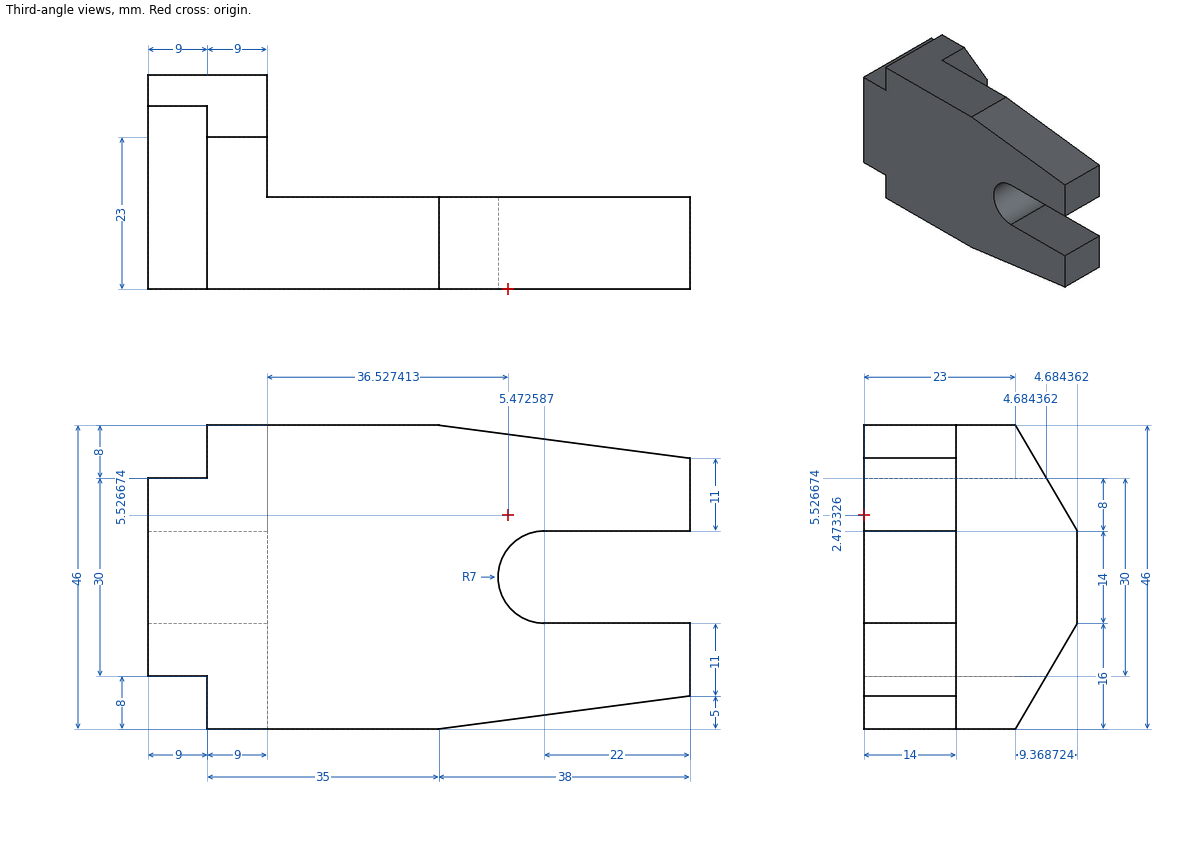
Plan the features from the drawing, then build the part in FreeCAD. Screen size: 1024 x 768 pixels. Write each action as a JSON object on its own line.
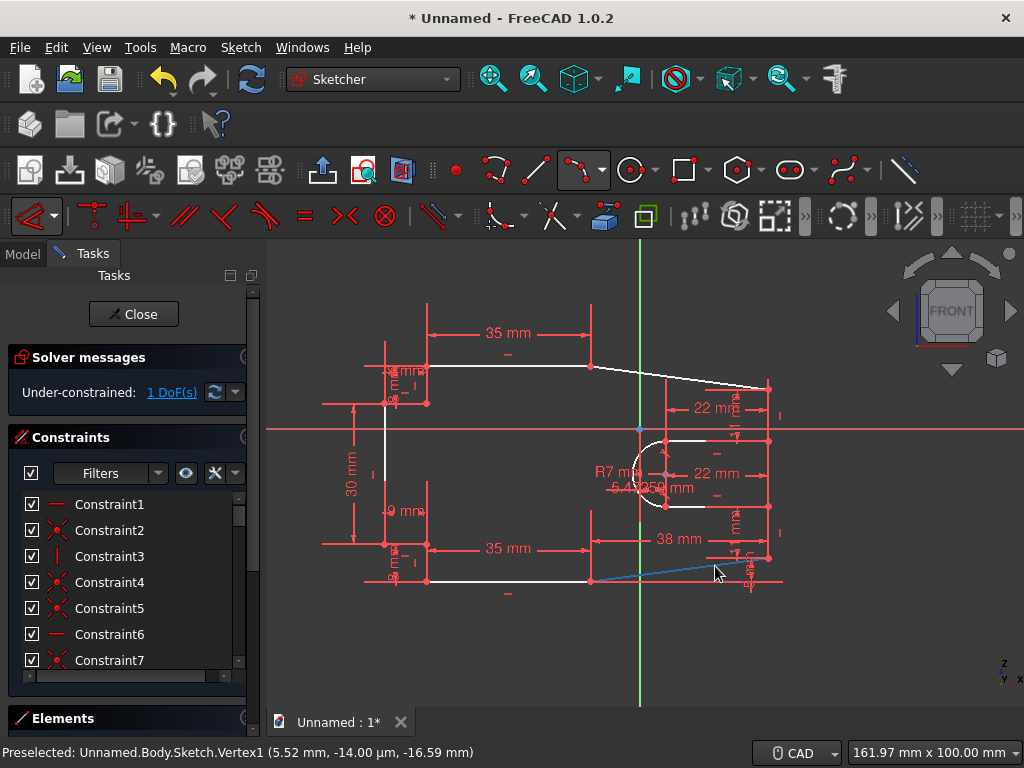
{"action": "scroll", "coordinate": [385, 404], "scroll_direction": "up", "scroll_amount": 3}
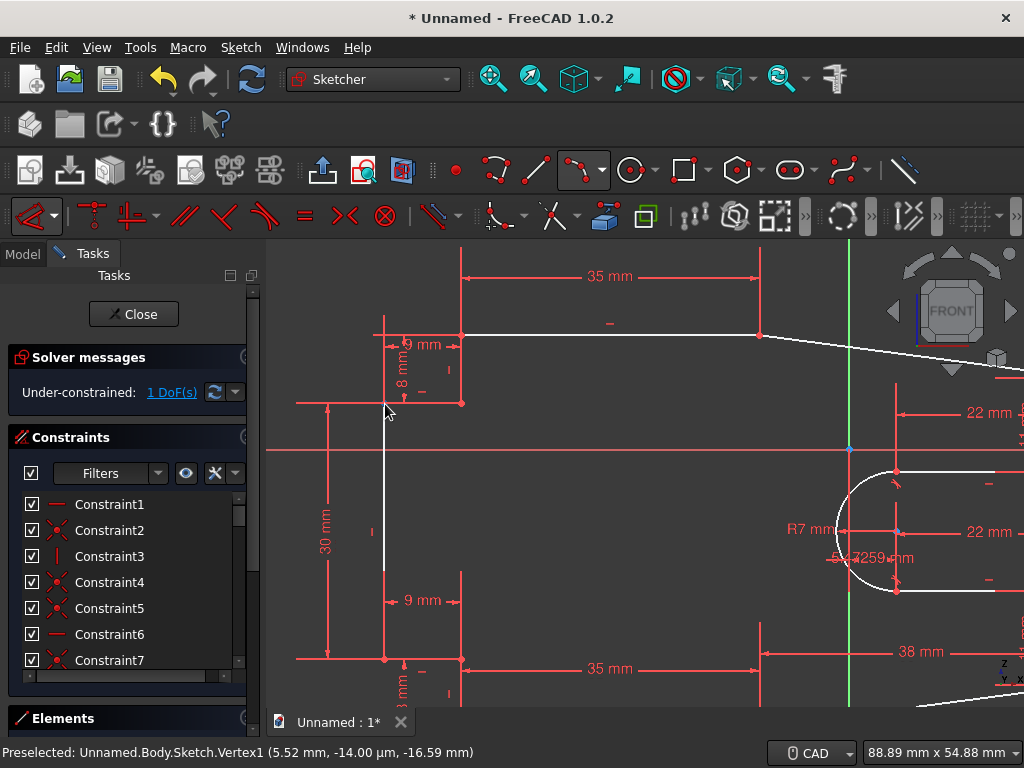
{"action": "left_click", "coordinate": [384, 403]}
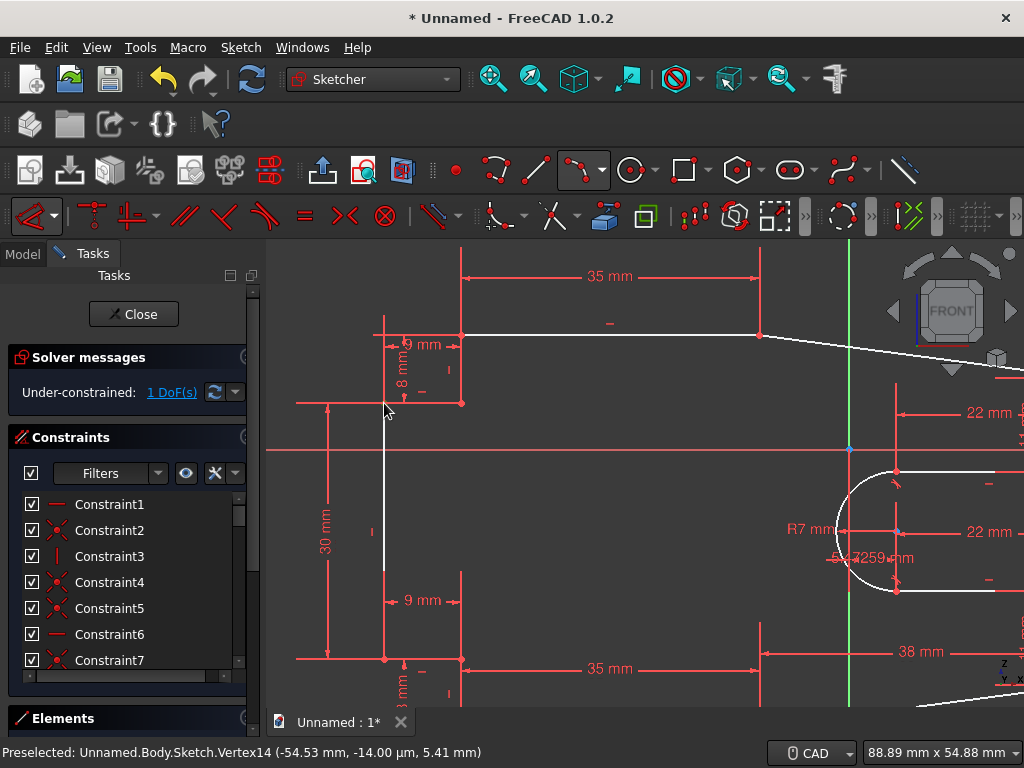
{"action": "key", "text": "i"}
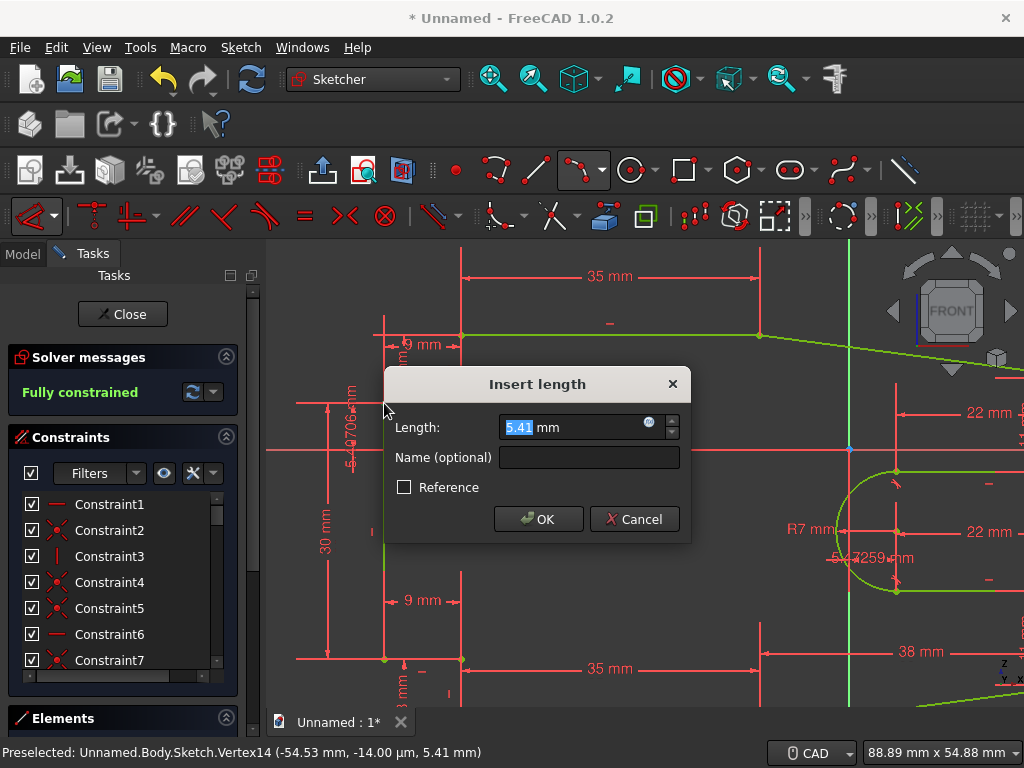
{"action": "type", "text": "5.526674"}
{"action": "key", "text": "Return"}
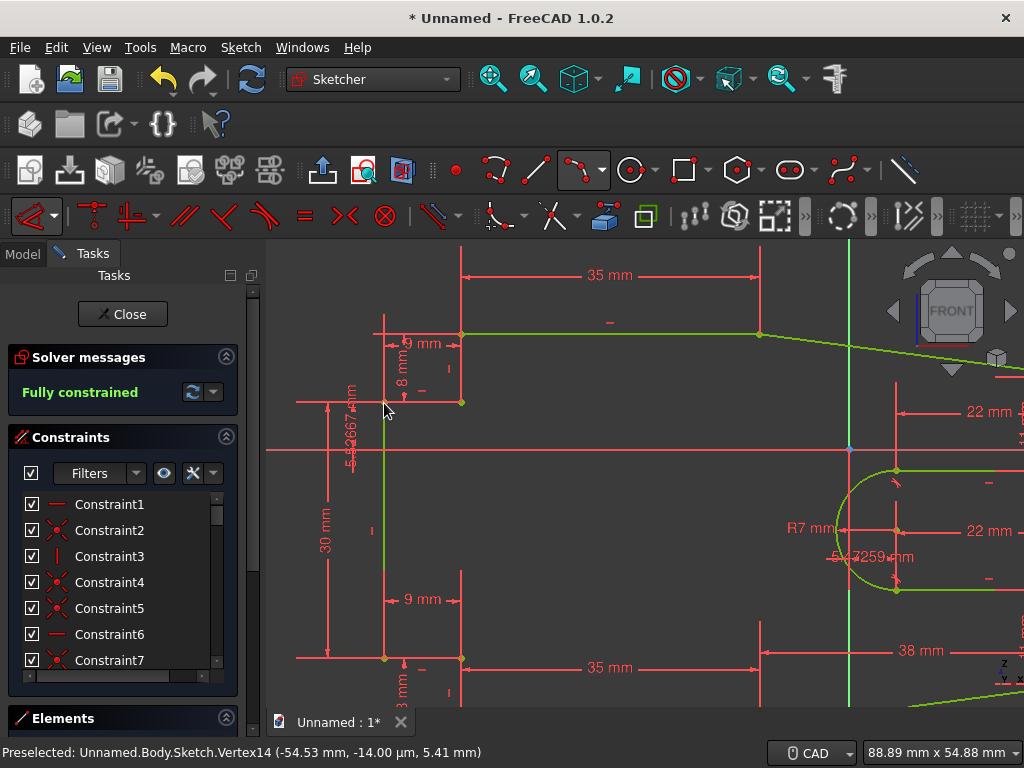
{"action": "left_click", "coordinate": [123, 314]}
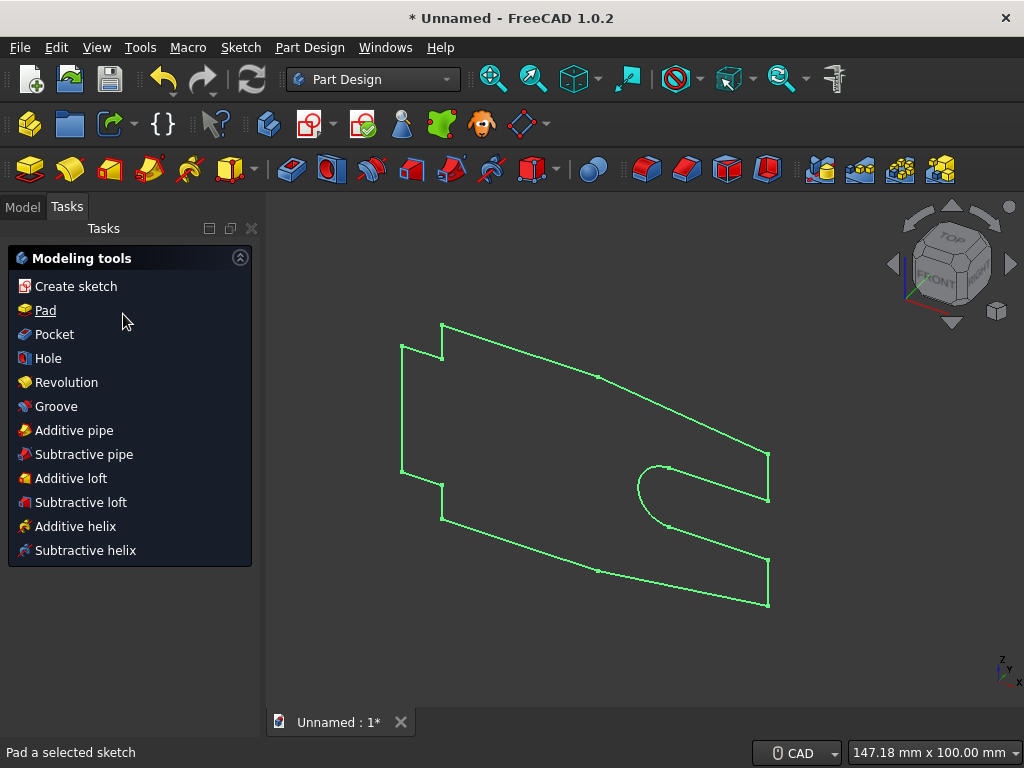
{"action": "left_click", "coordinate": [30, 170]}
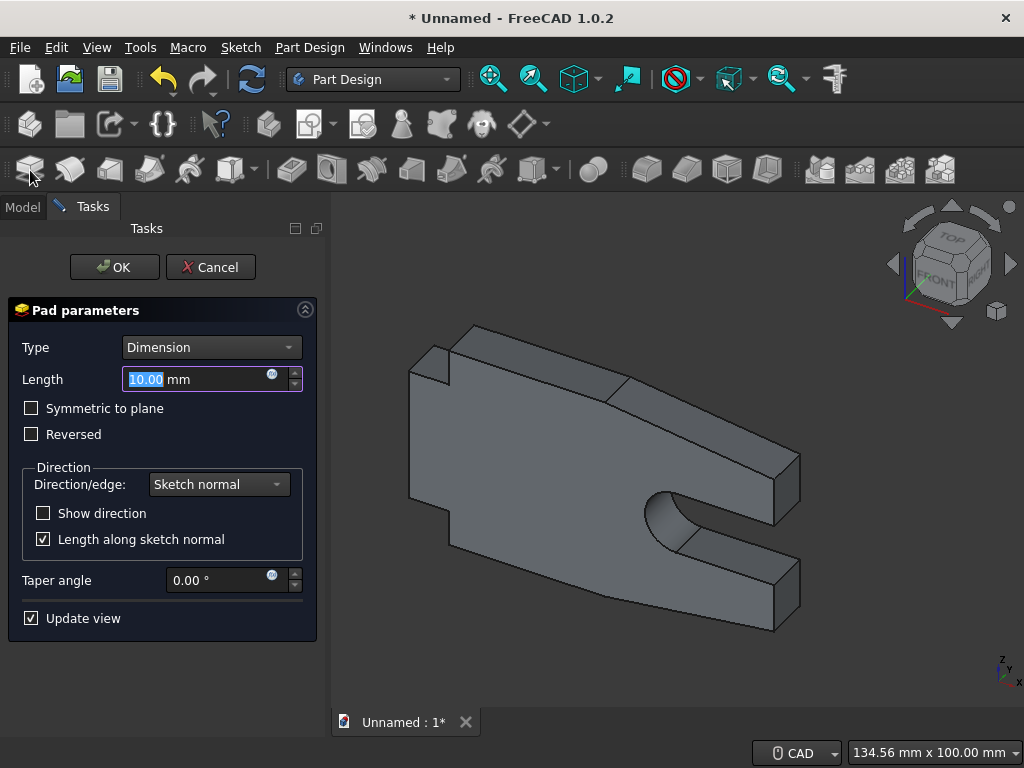
{"action": "type", "text": "14"}
{"action": "key", "text": "Tab"}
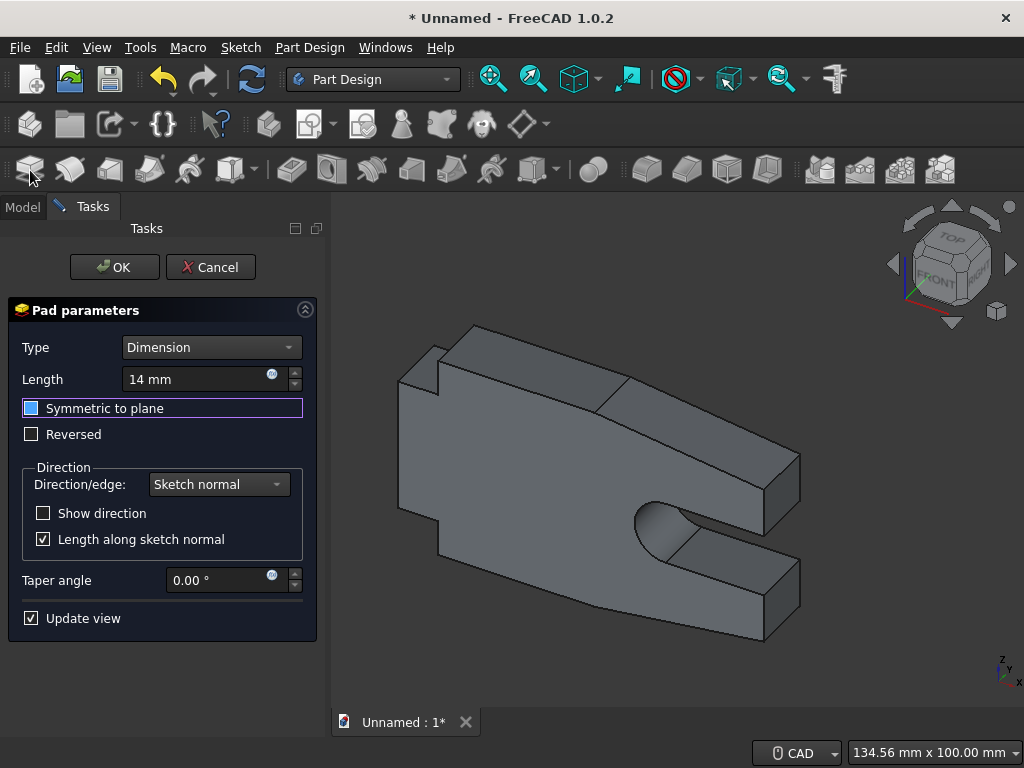
{"action": "left_click", "coordinate": [30, 434]}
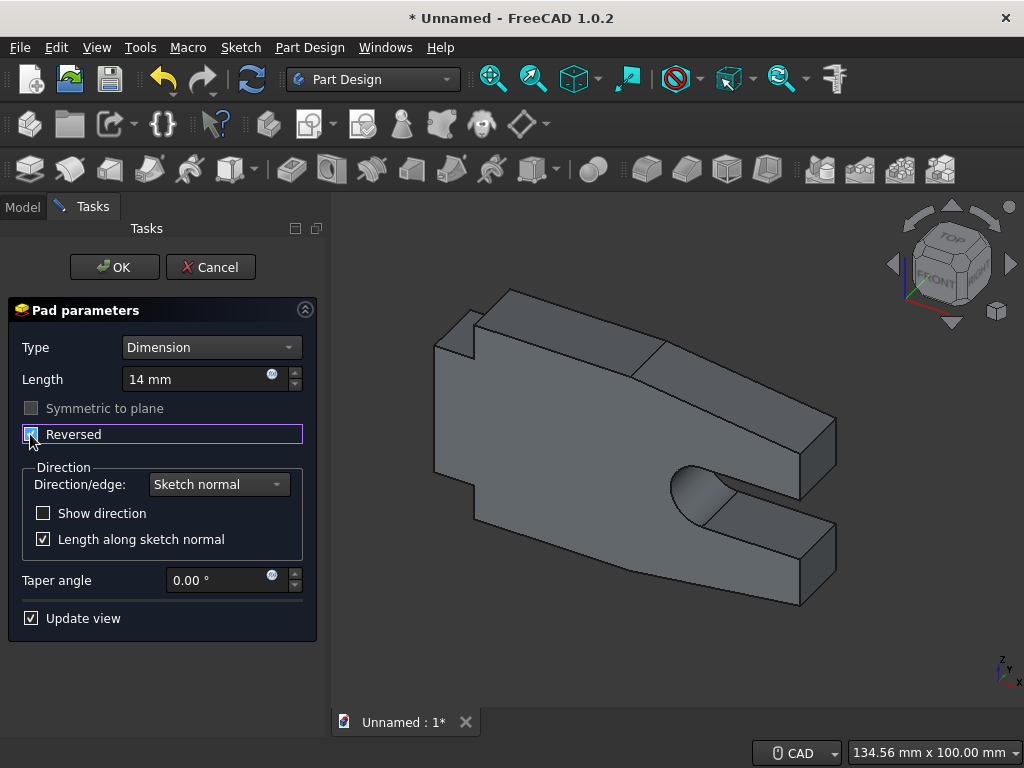
{"action": "left_click", "coordinate": [115, 267]}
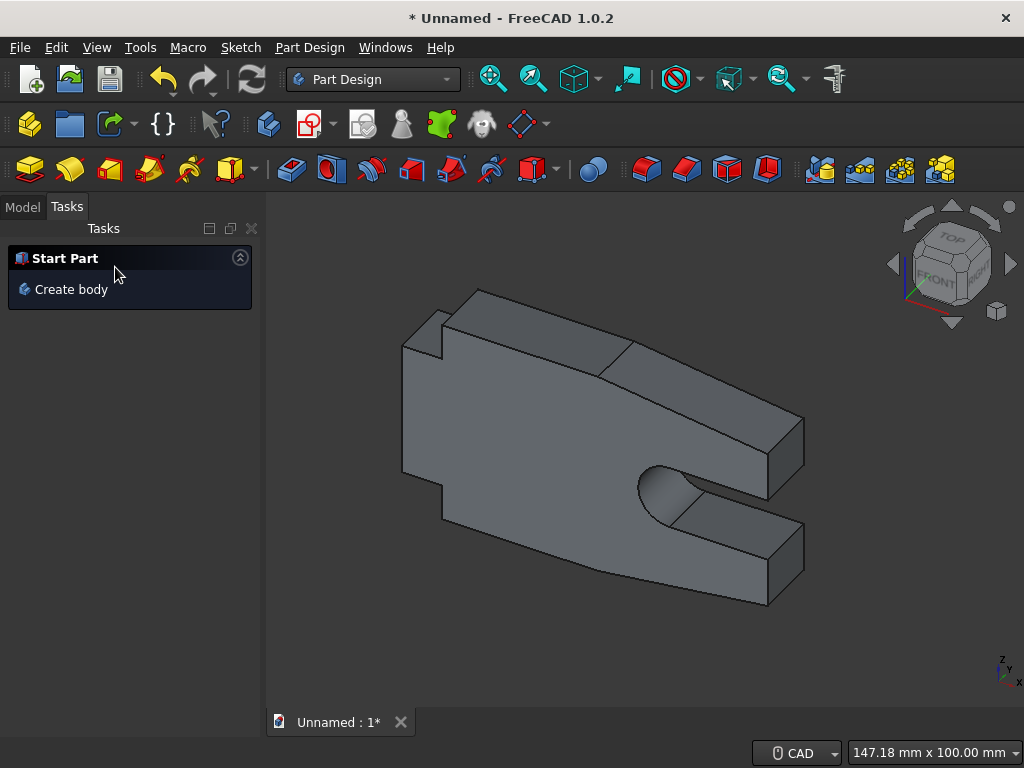
{"action": "left_click", "coordinate": [310, 124]}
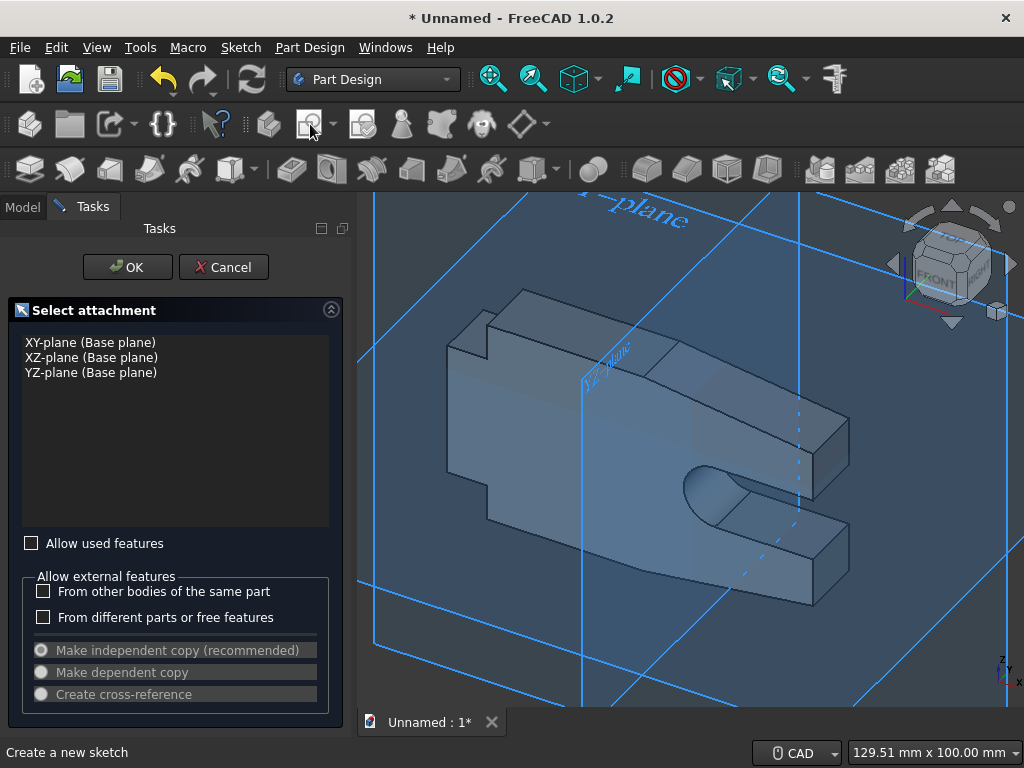
{"action": "left_click", "coordinate": [82, 358]}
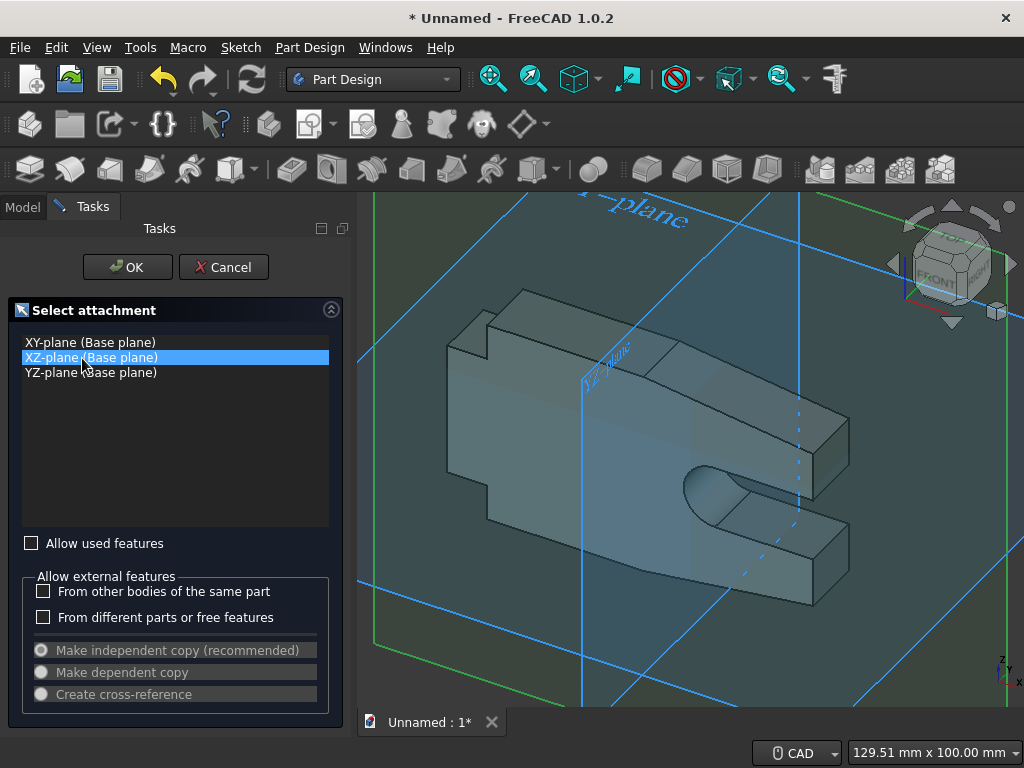
{"action": "left_click", "coordinate": [128, 267]}